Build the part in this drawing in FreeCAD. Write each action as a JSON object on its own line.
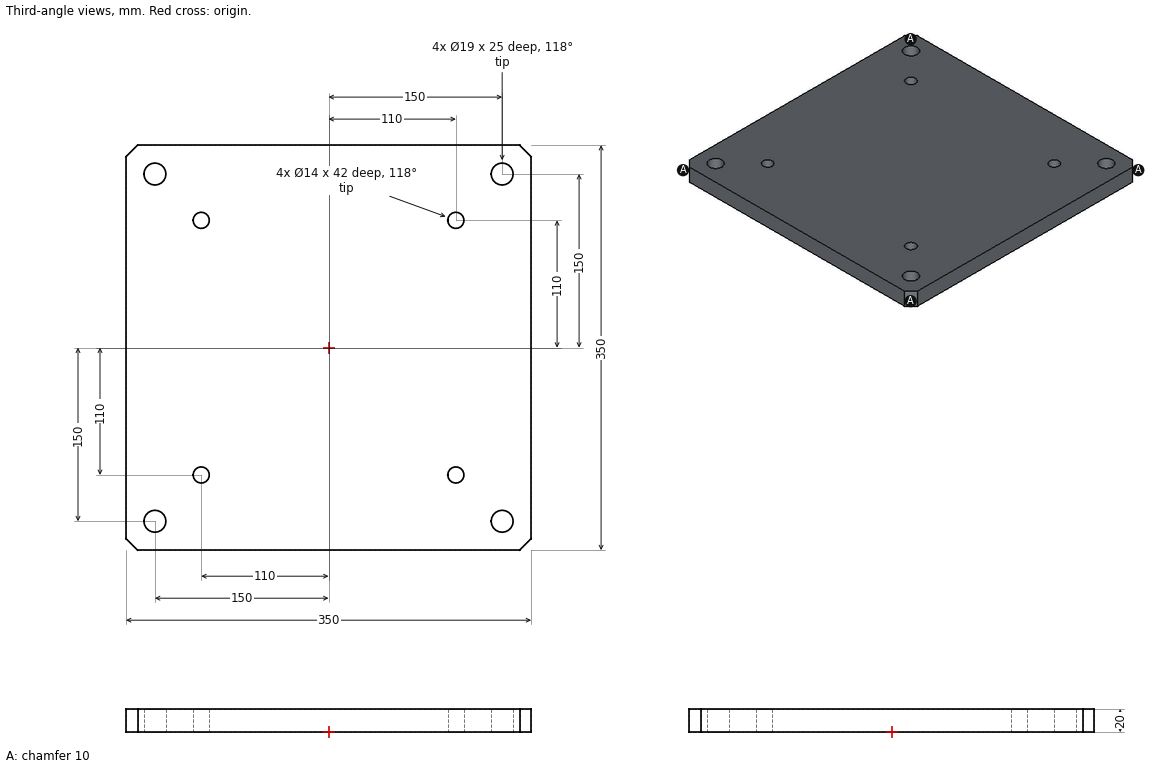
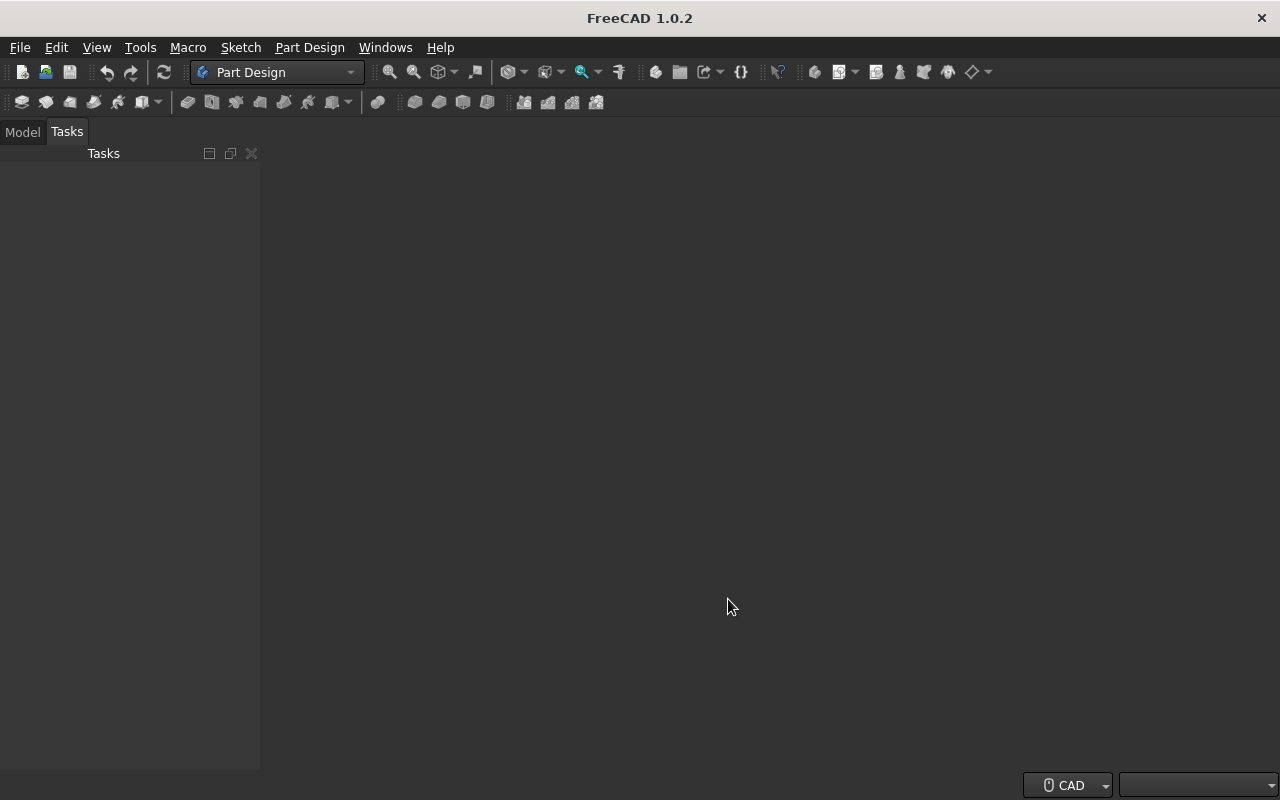
{"action": "left_click", "coordinate": [22, 72]}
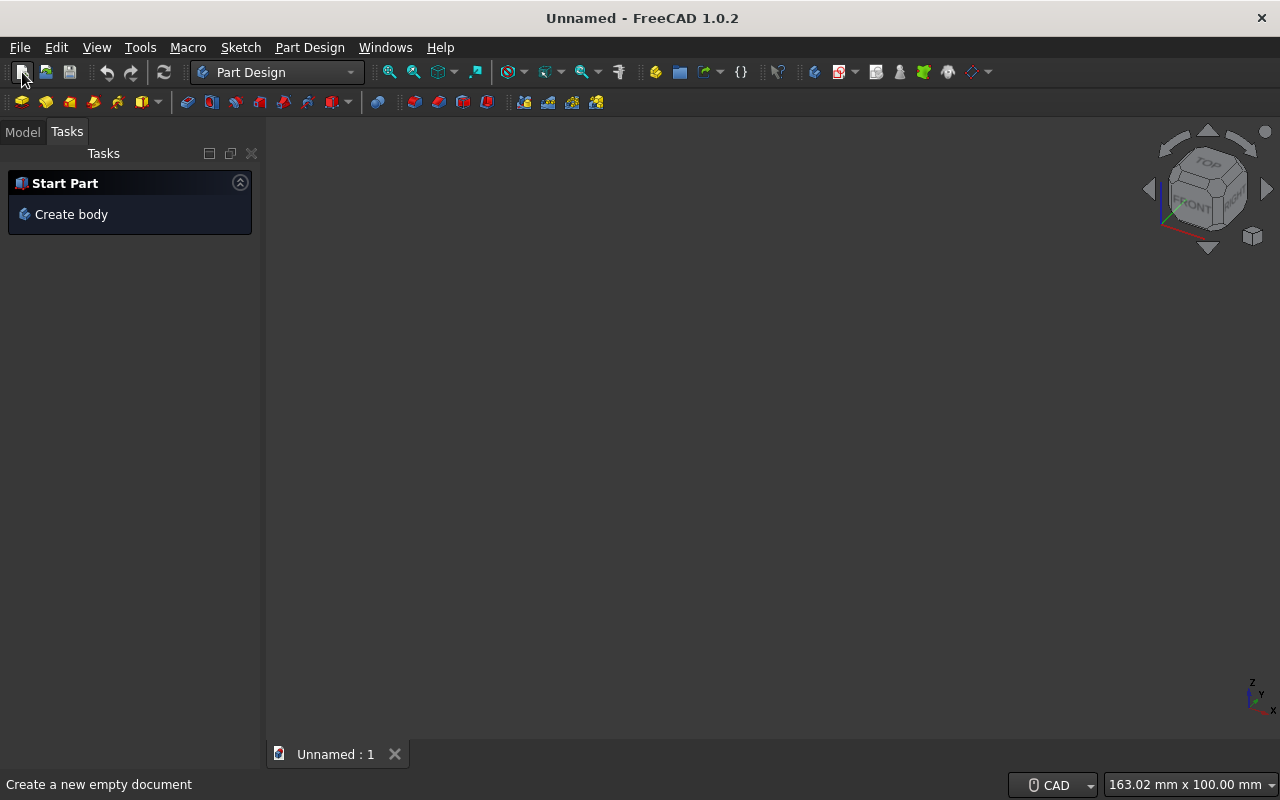
{"action": "left_click", "coordinate": [840, 72]}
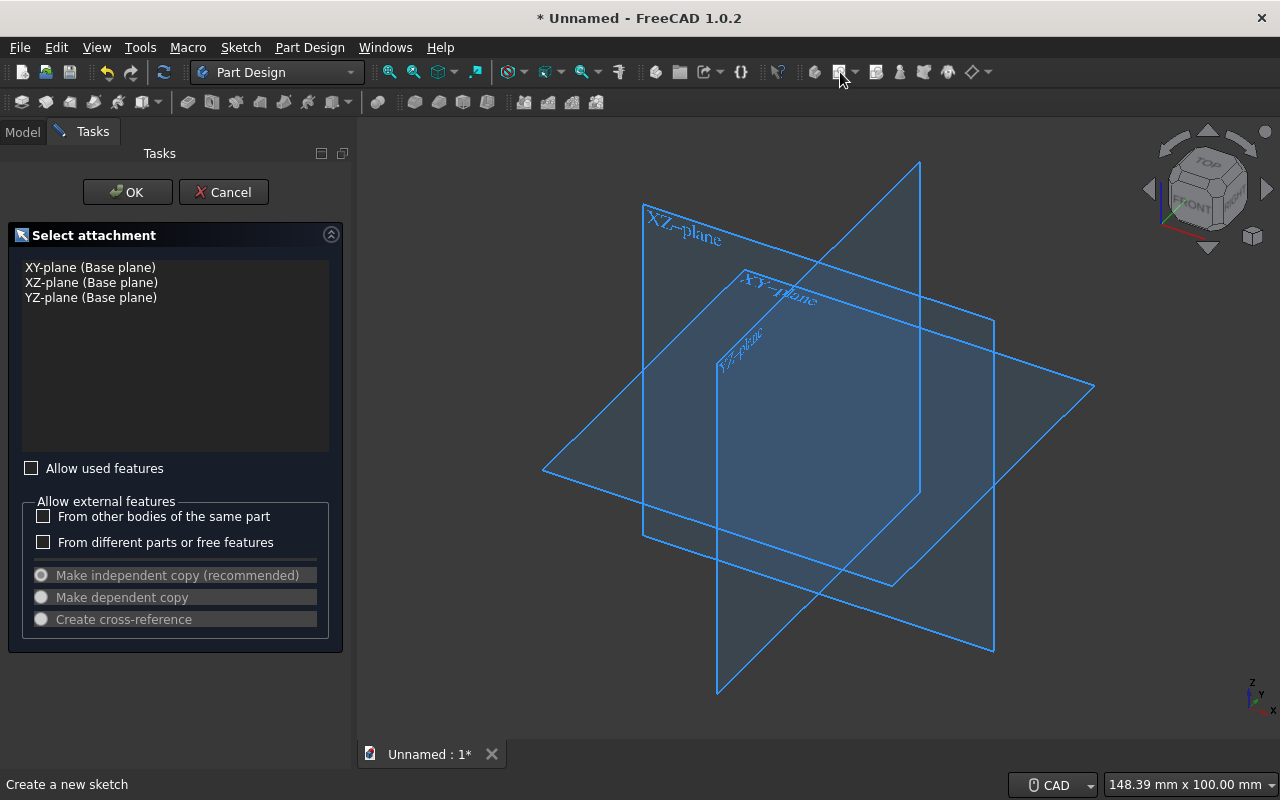
{"action": "left_click", "coordinate": [82, 268]}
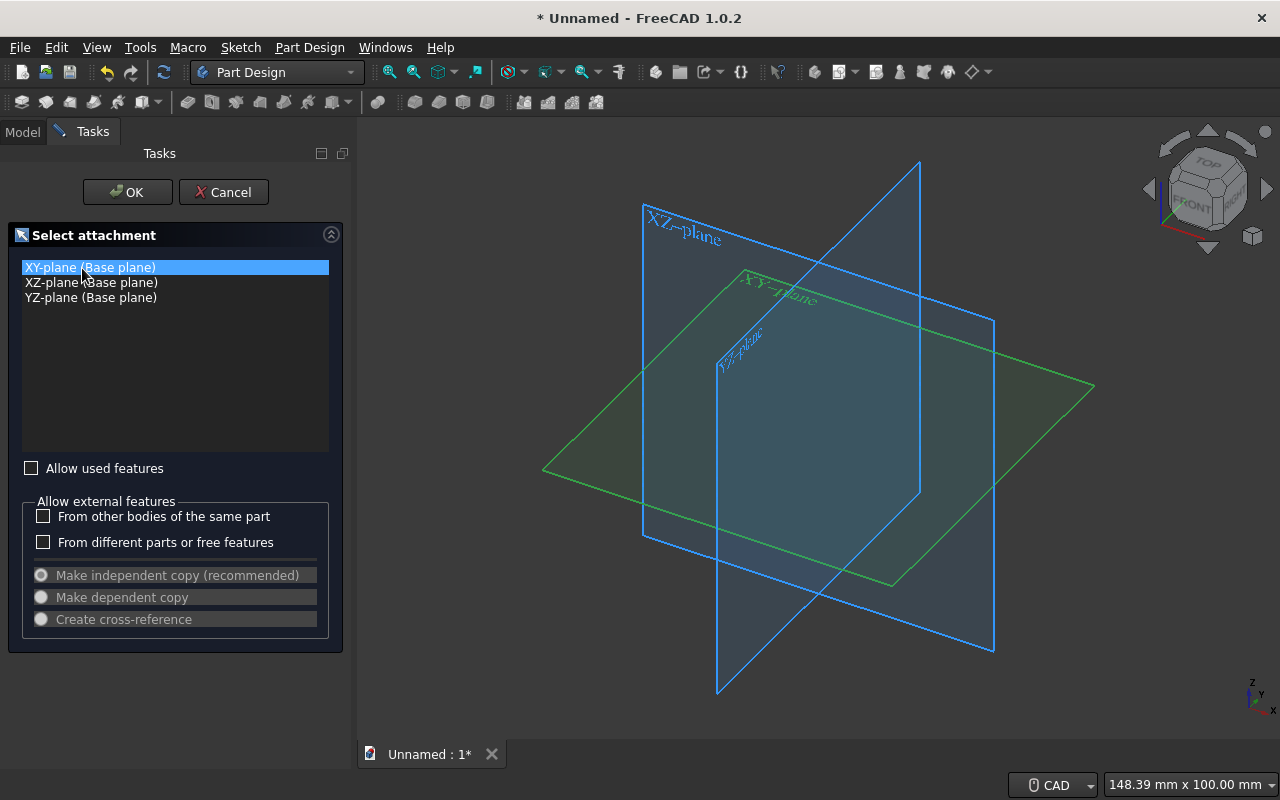
{"action": "left_click", "coordinate": [128, 192]}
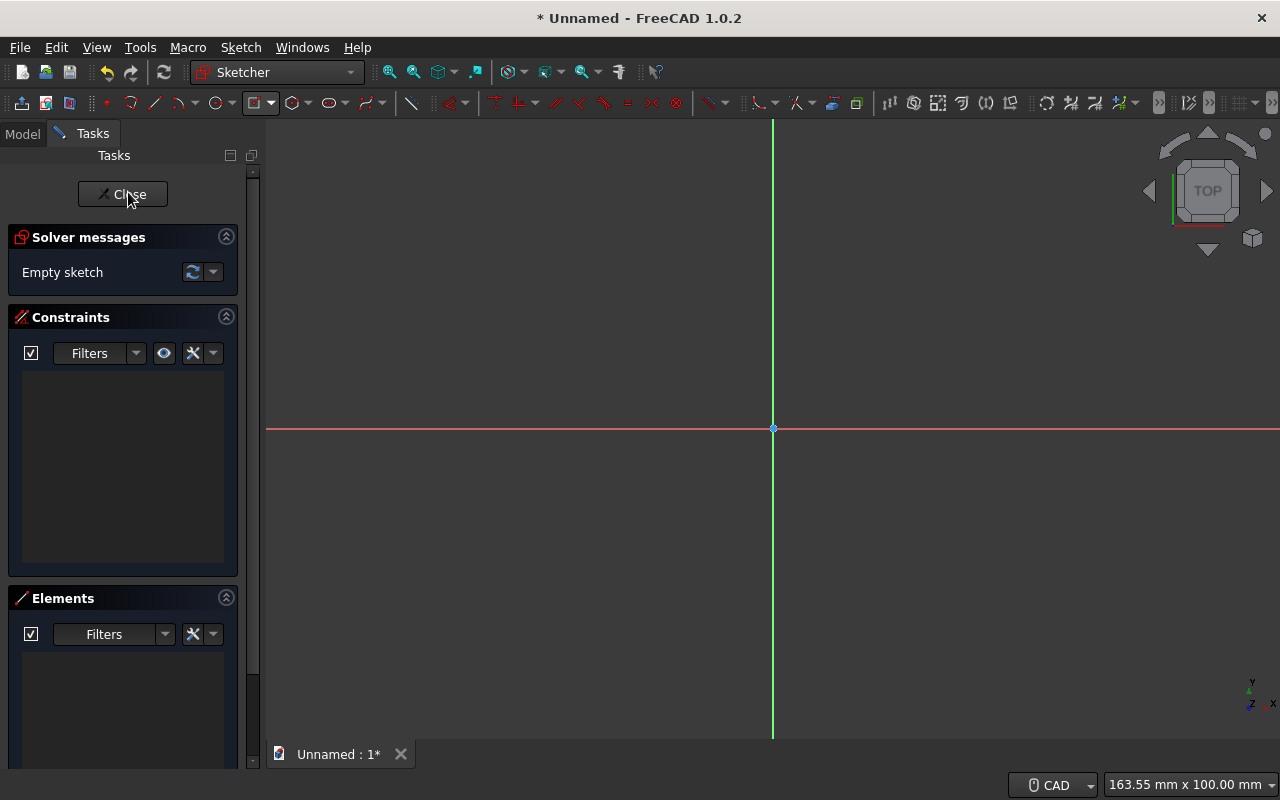
{"action": "scroll", "coordinate": [687, 429], "scroll_direction": "down", "scroll_amount": 8}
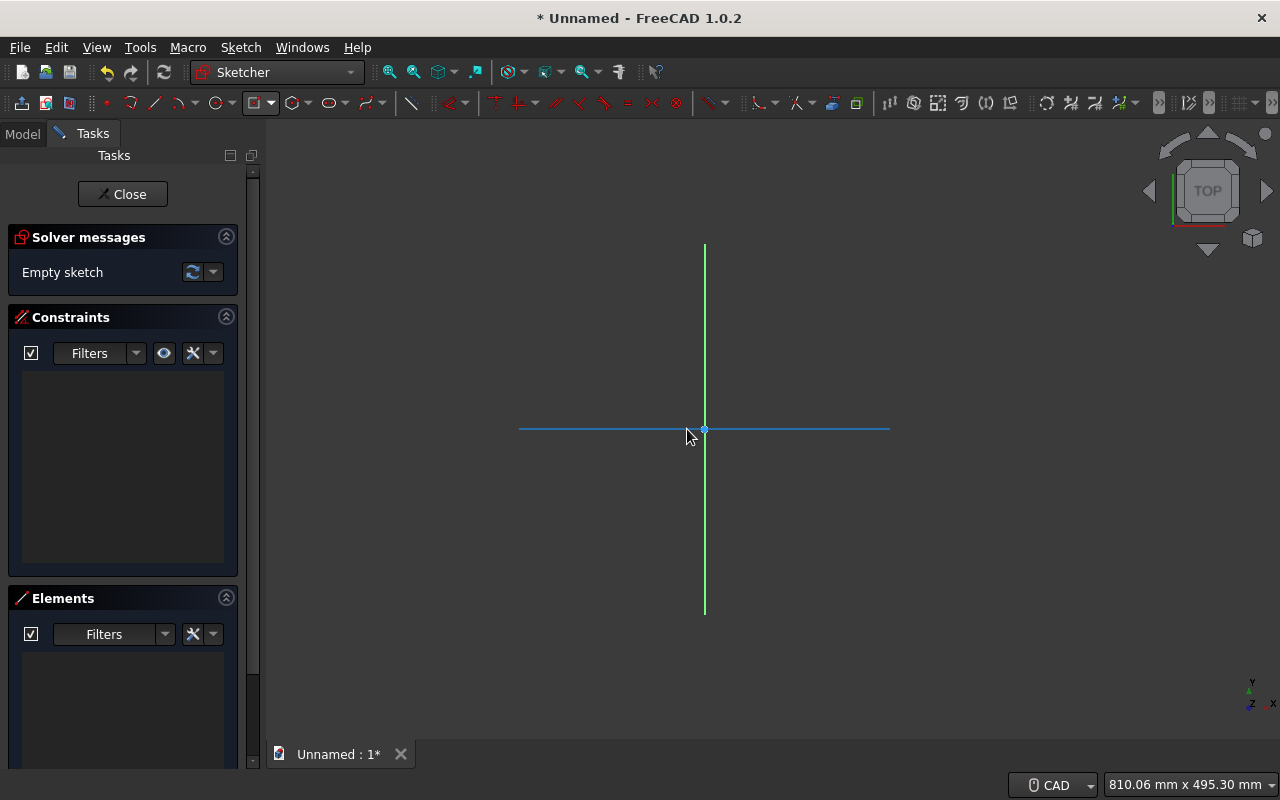
{"action": "left_click", "coordinate": [254, 104]}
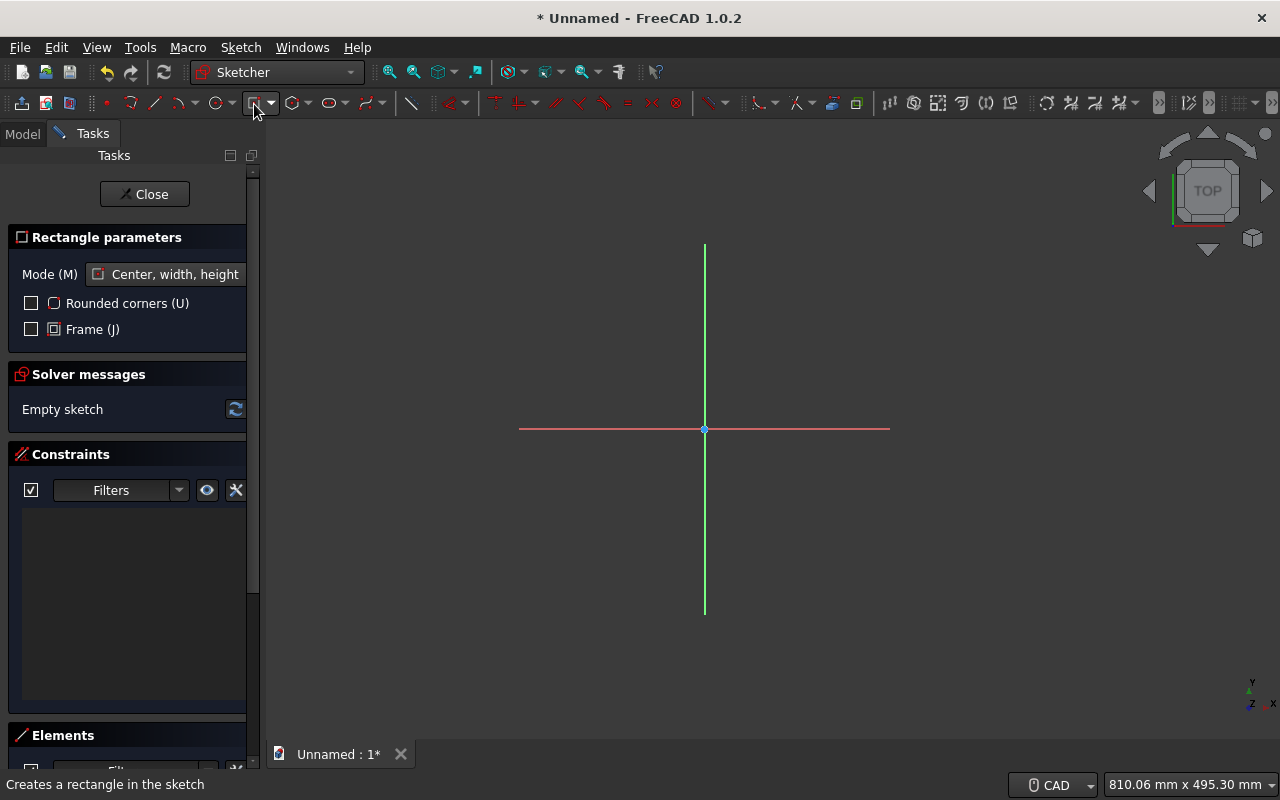
{"action": "left_click", "coordinate": [705, 429]}
{"action": "mouse_move", "coordinate": [924, 210]}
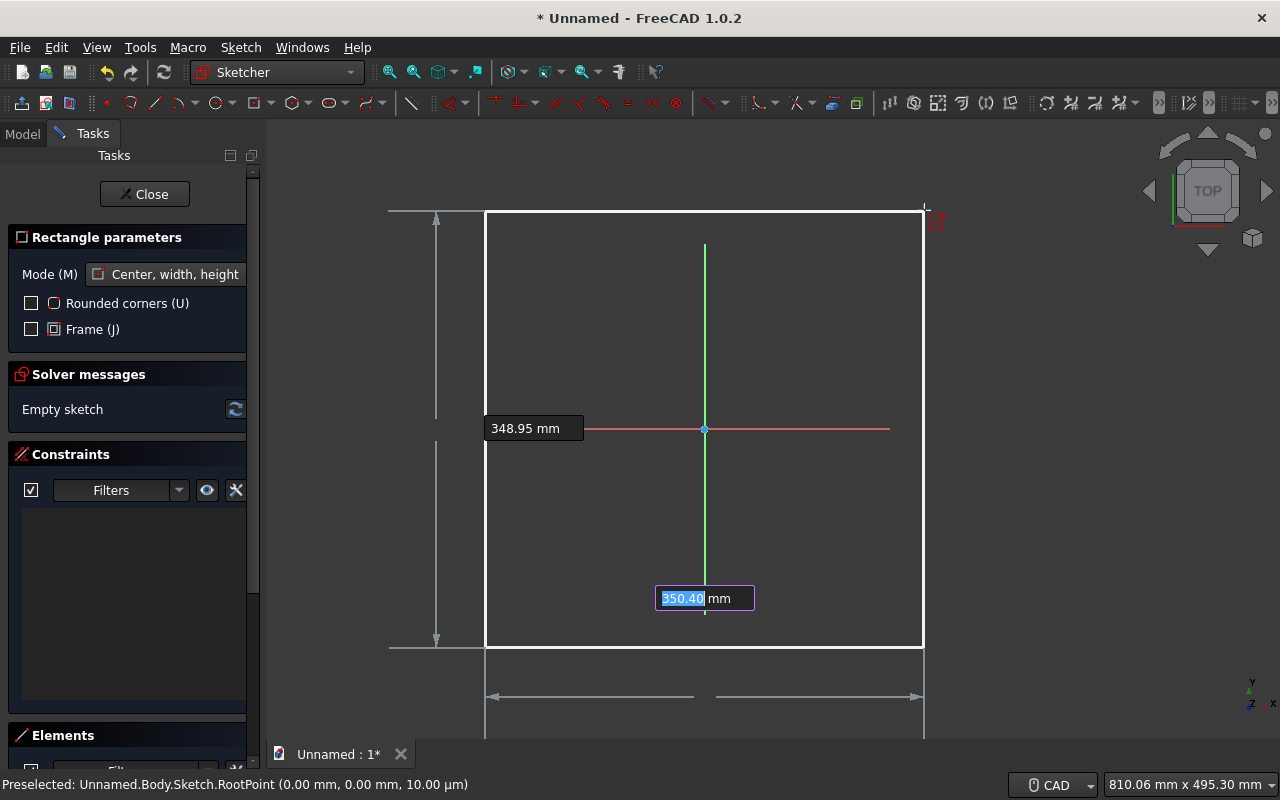
{"action": "type", "text": "350"}
{"action": "key", "text": "Tab"}
{"action": "type", "text": "350"}
{"action": "key", "text": "Return"}
{"action": "key", "text": "Escape"}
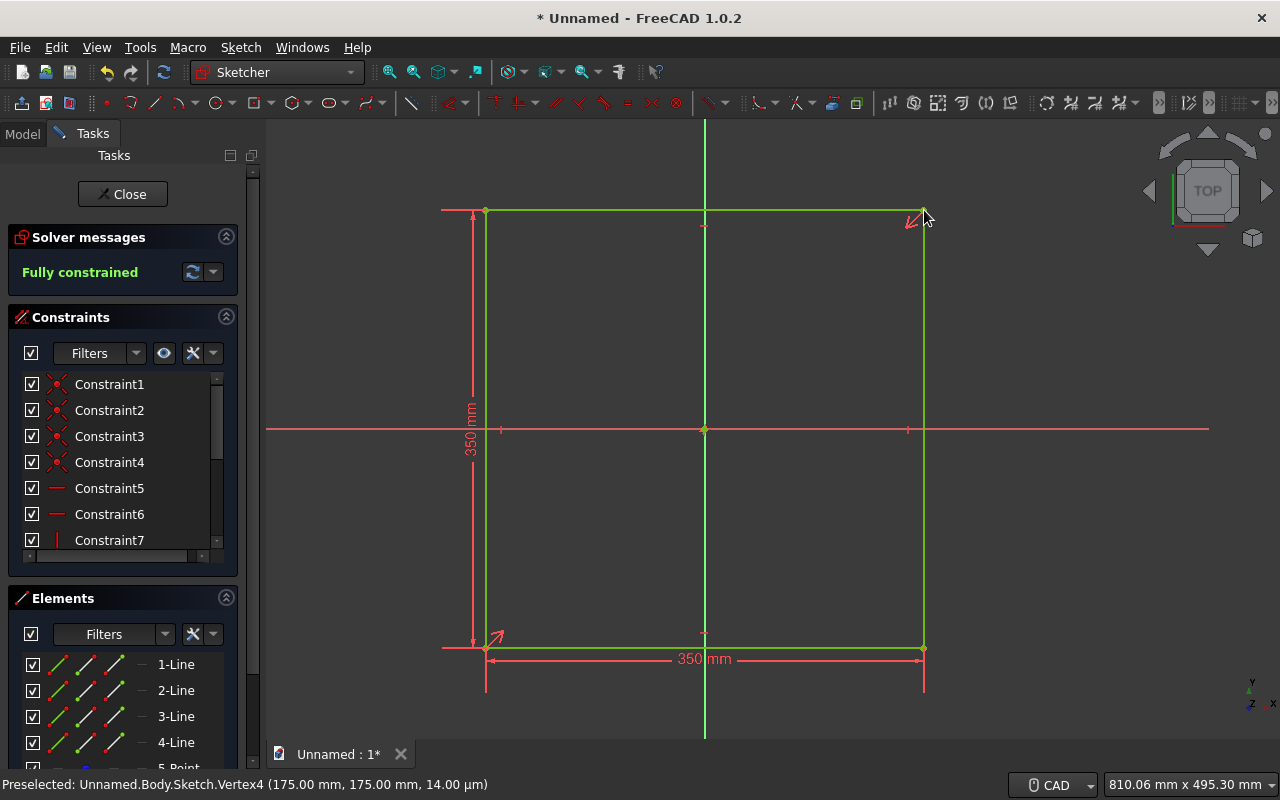
{"action": "left_click", "coordinate": [123, 194]}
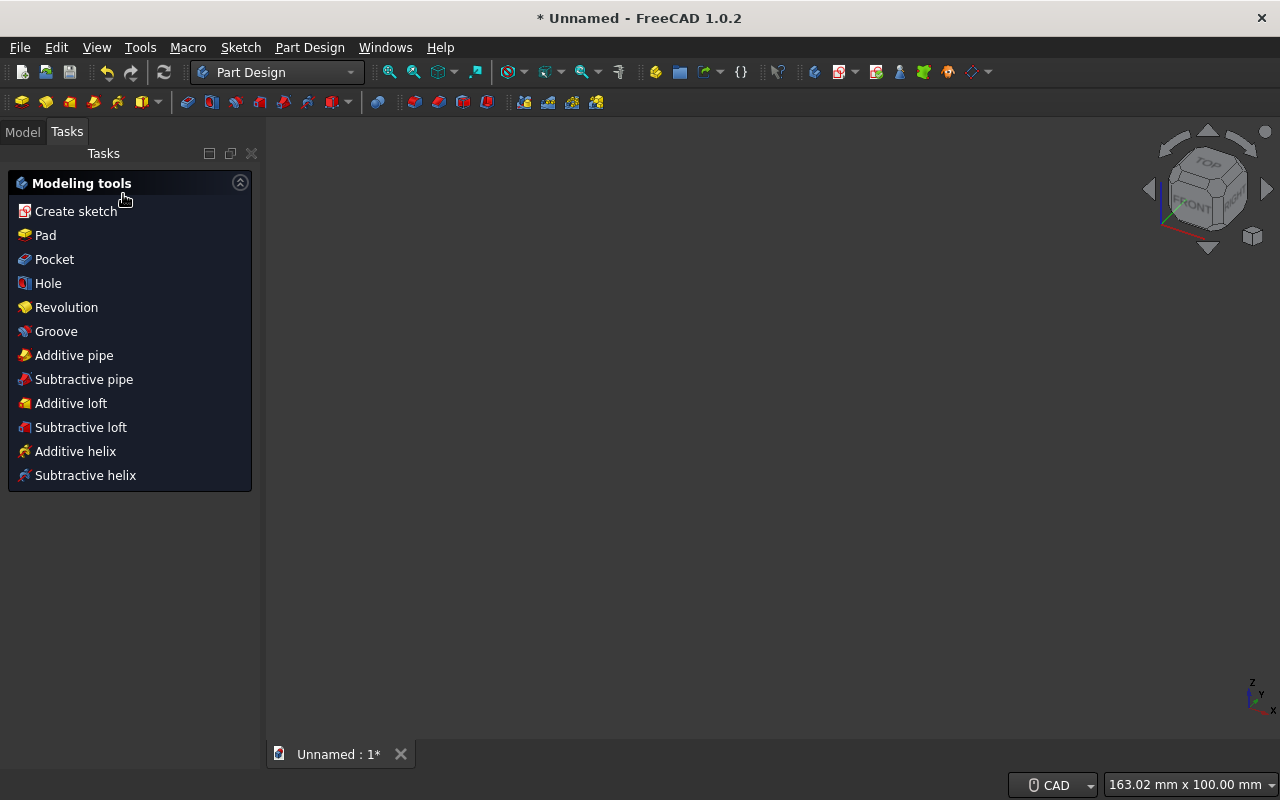
{"action": "left_click", "coordinate": [22, 102]}